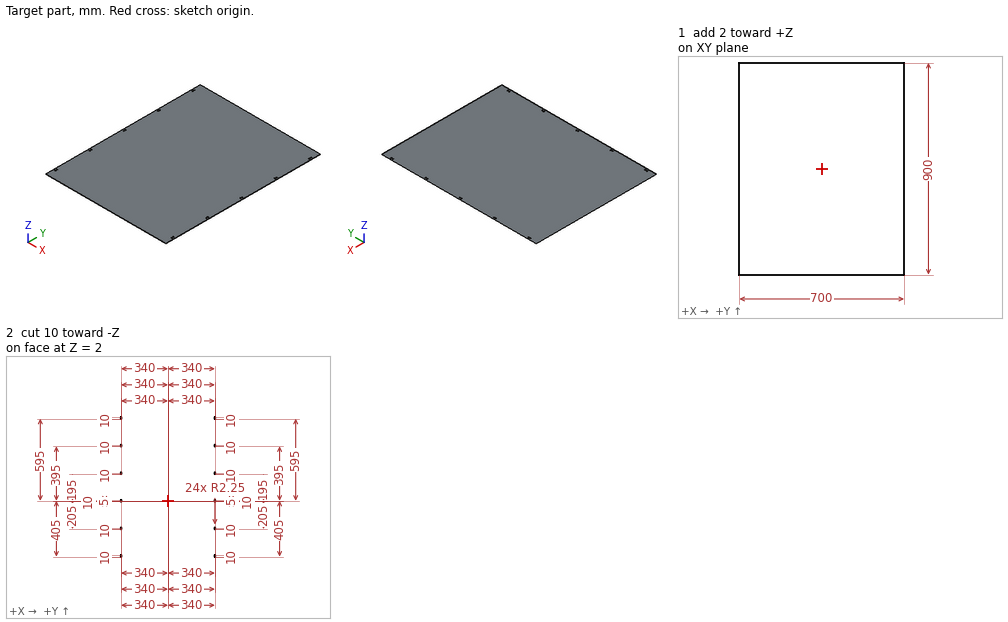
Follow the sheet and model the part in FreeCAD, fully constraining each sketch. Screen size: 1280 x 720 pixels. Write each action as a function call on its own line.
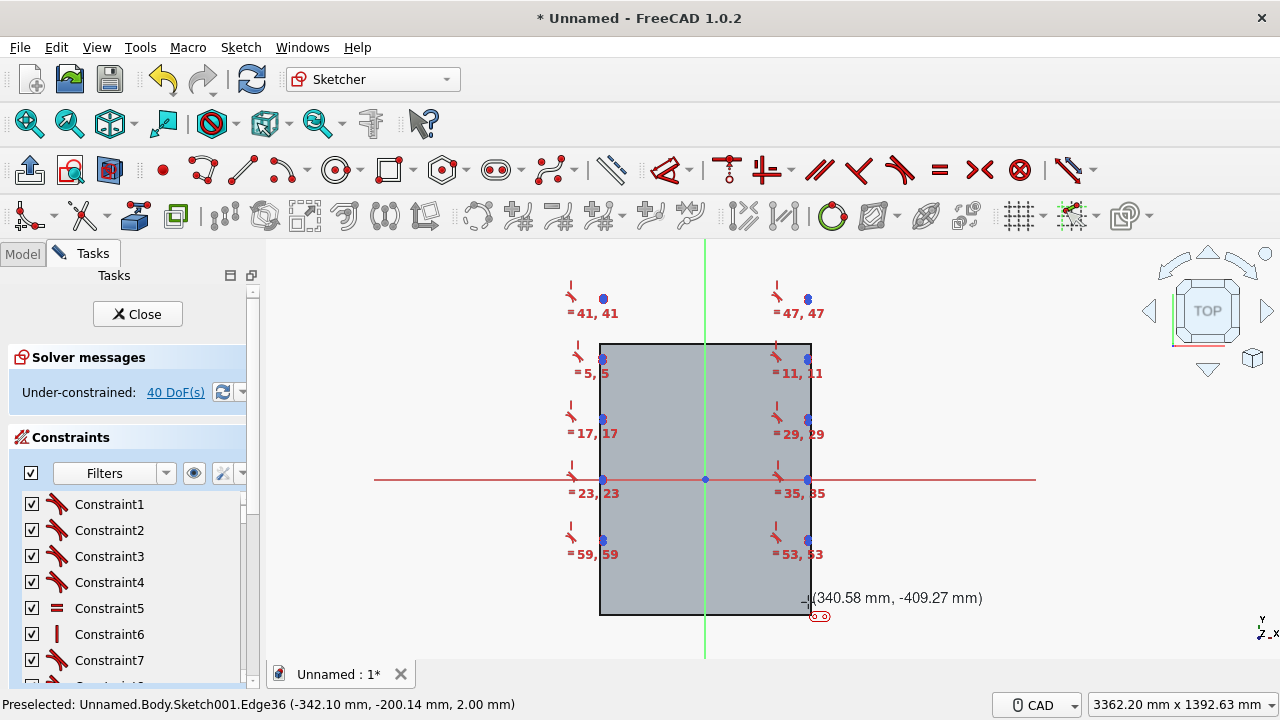
click(808, 602)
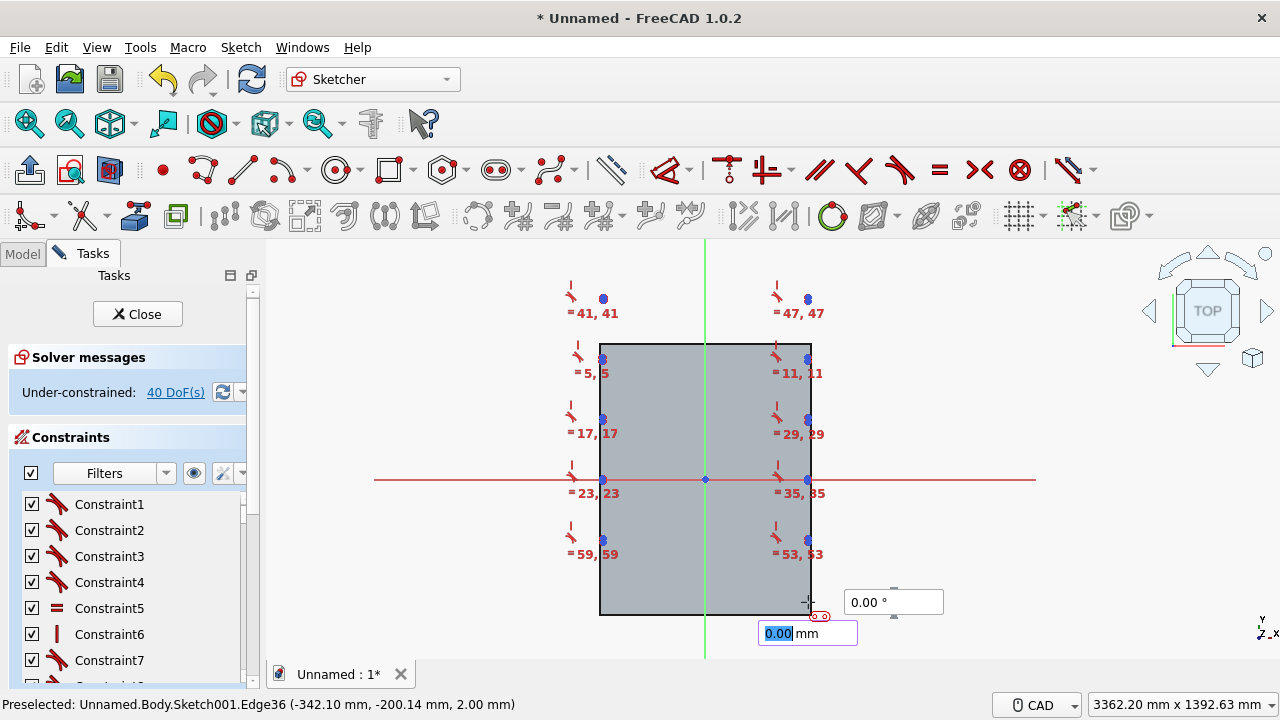
scroll(808, 599, up, 9)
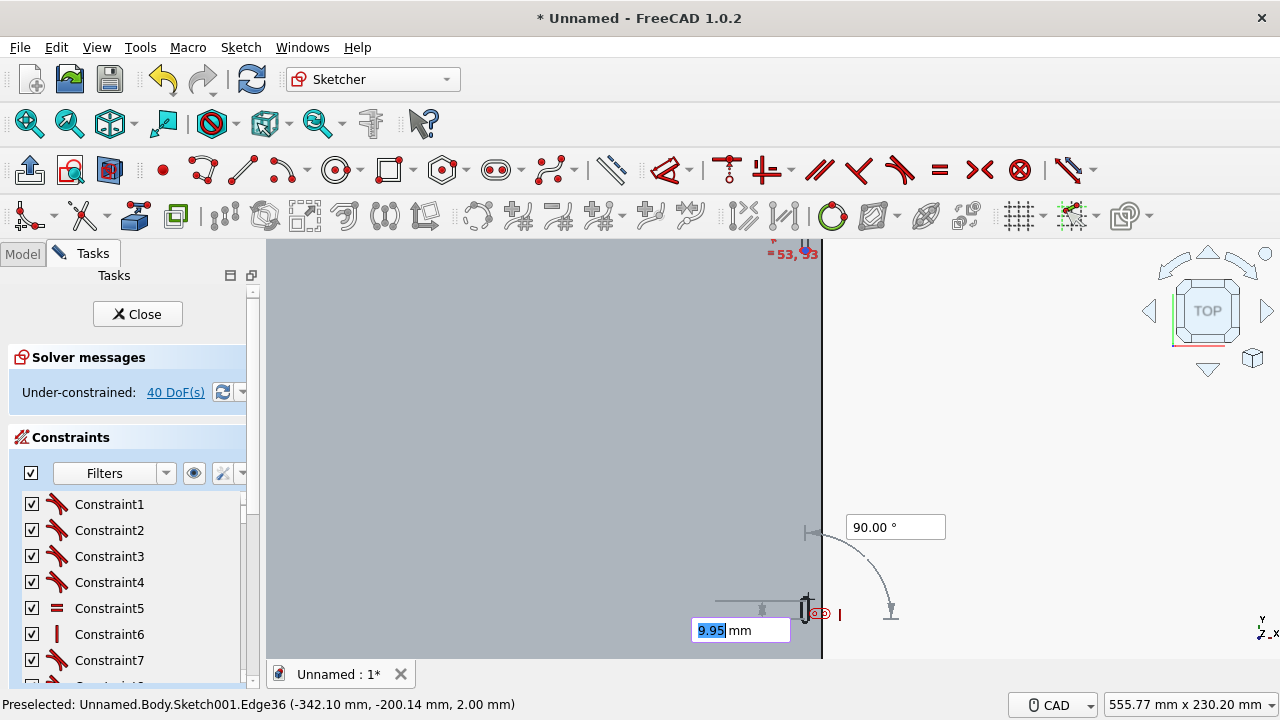
click(805, 593)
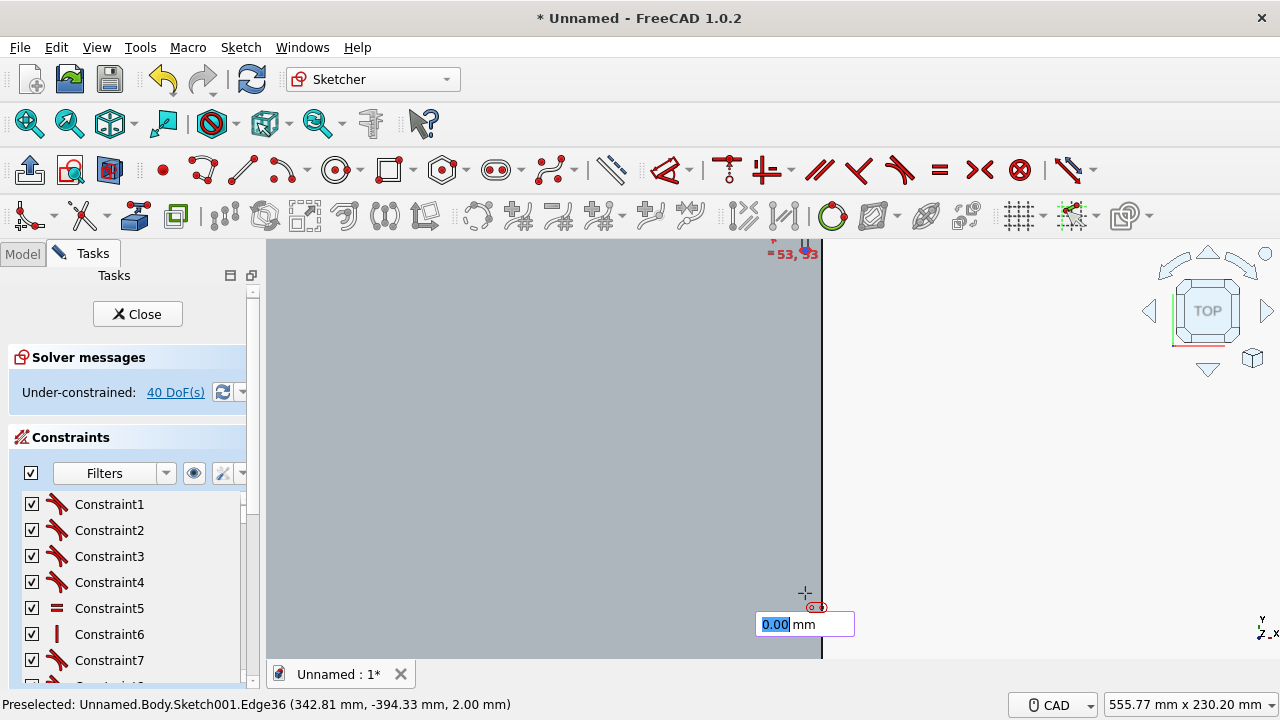
scroll(800, 602, up, 7)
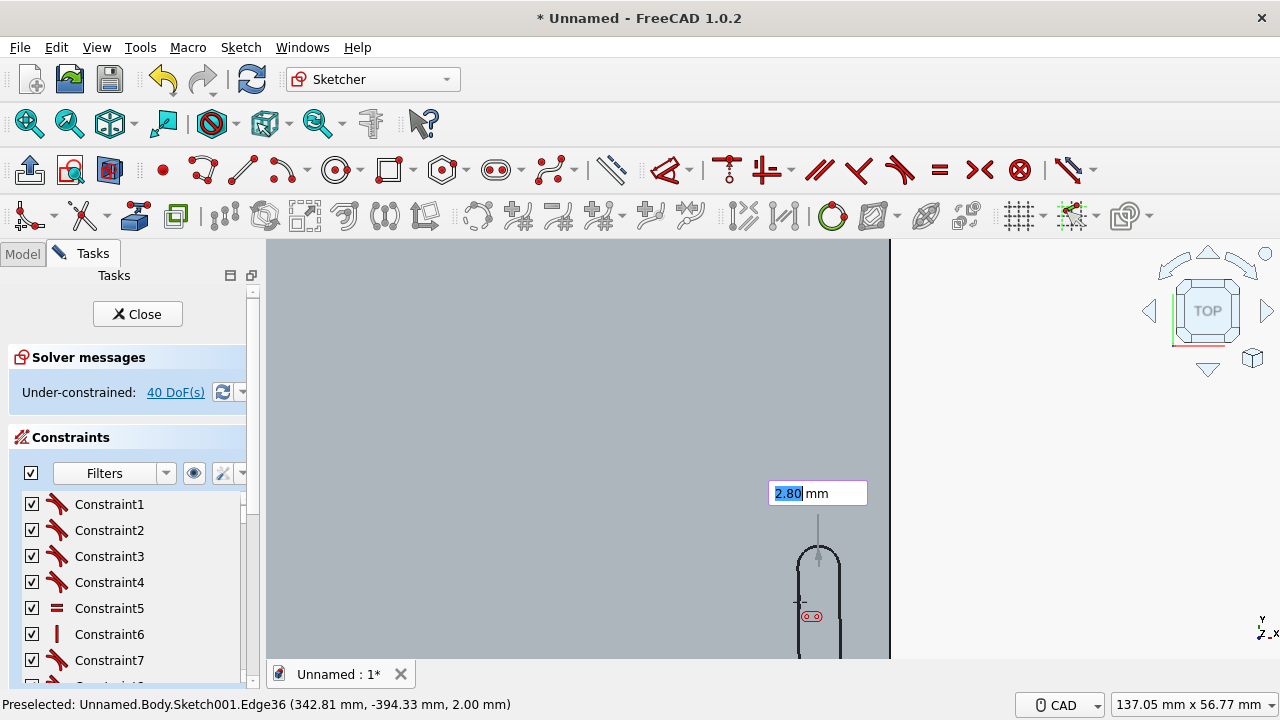
click(799, 599)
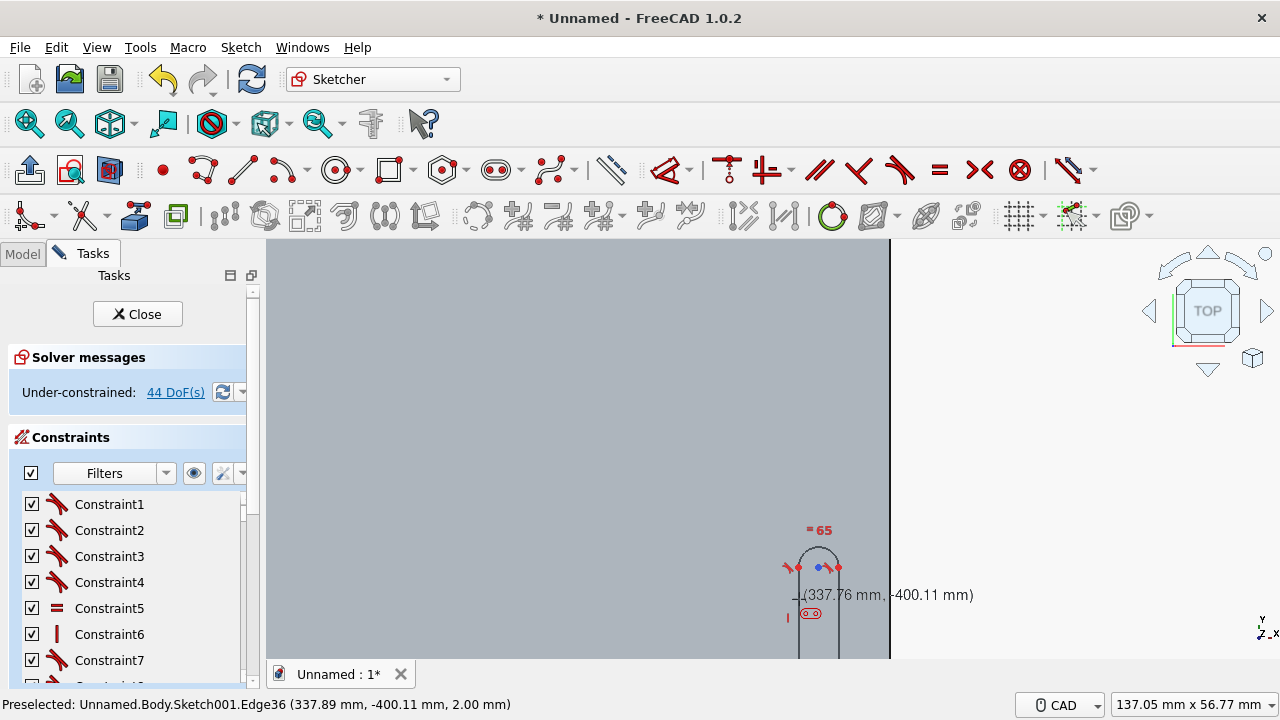
scroll(807, 600, down, 16)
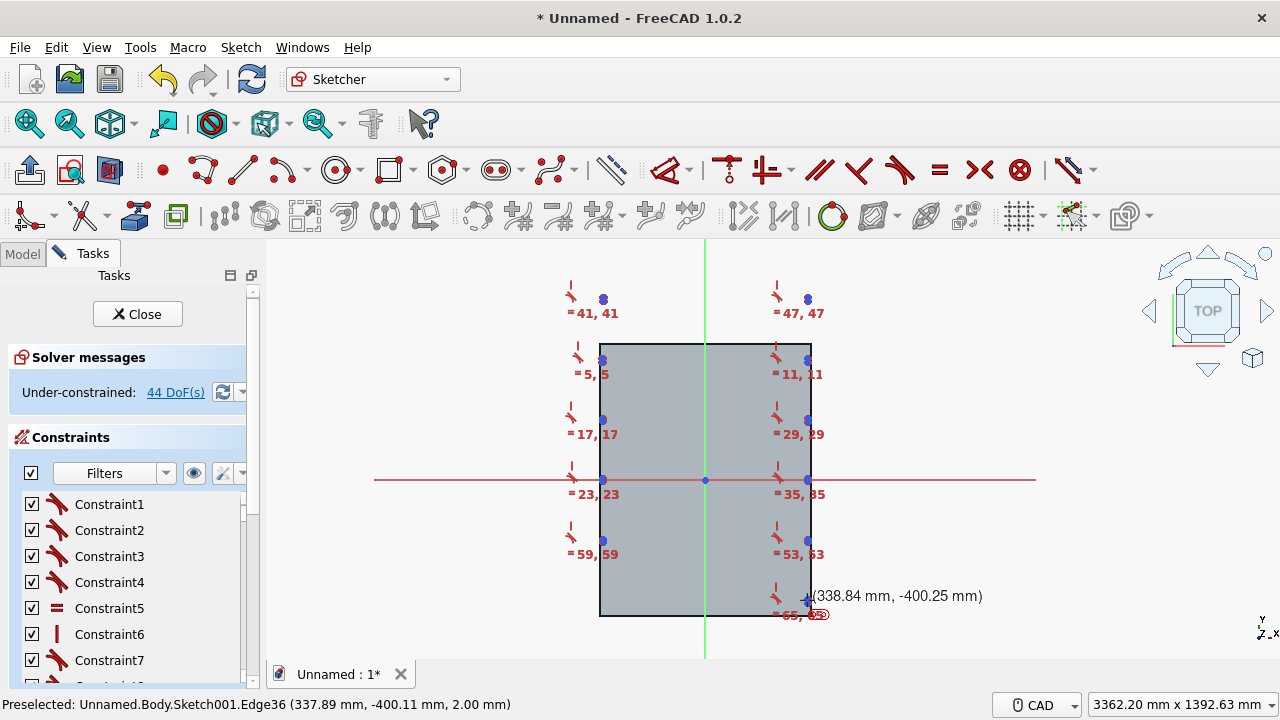
scroll(603, 602, up, 18)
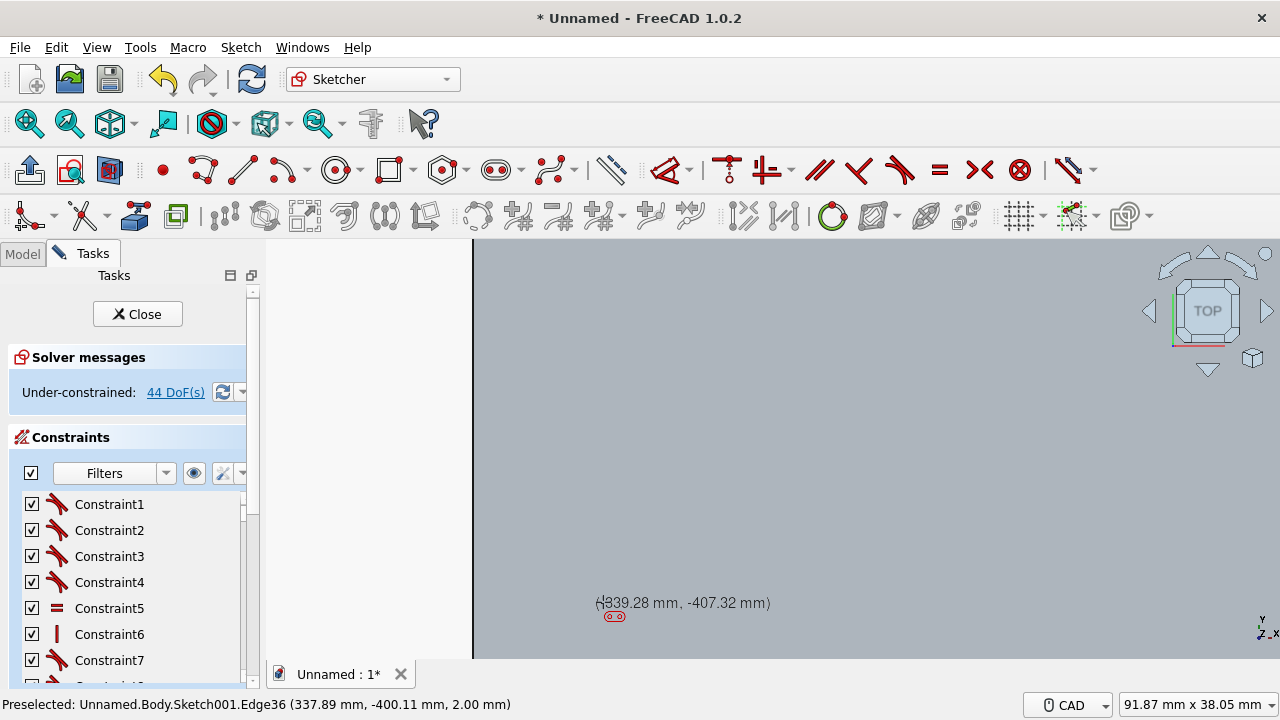
scroll(602, 602, down, 18)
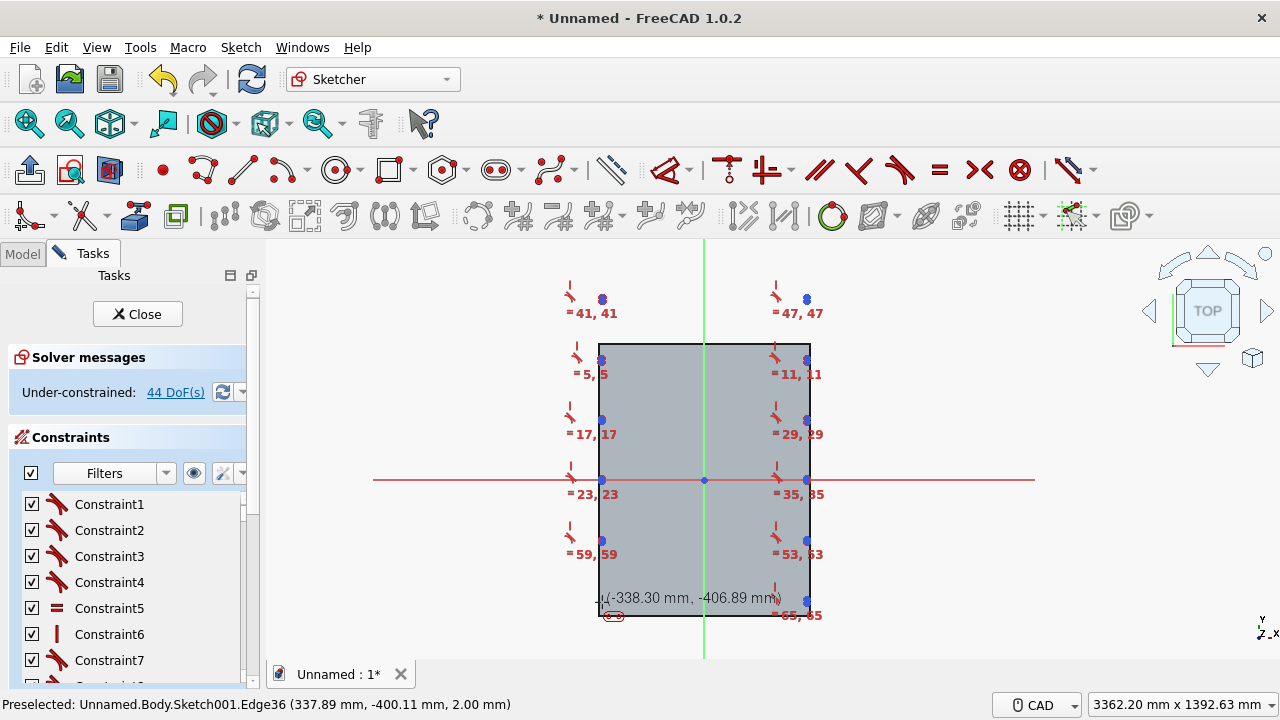
click(602, 602)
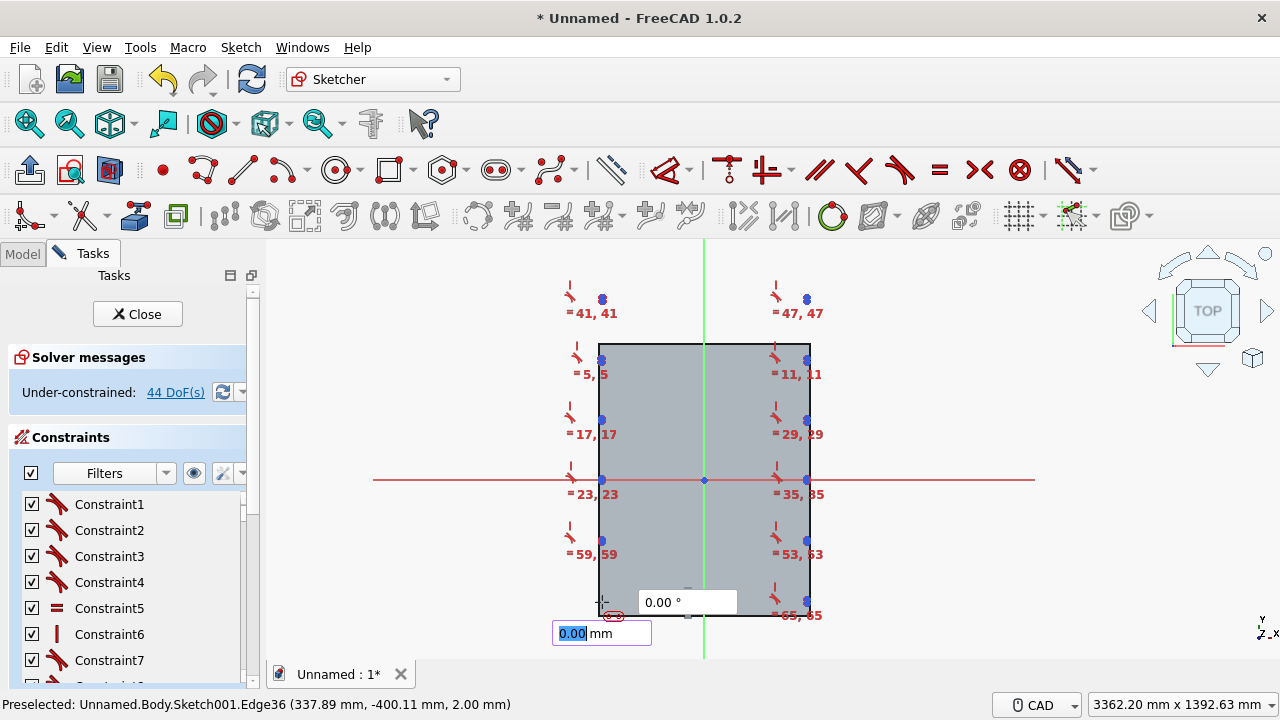
scroll(602, 599, up, 9)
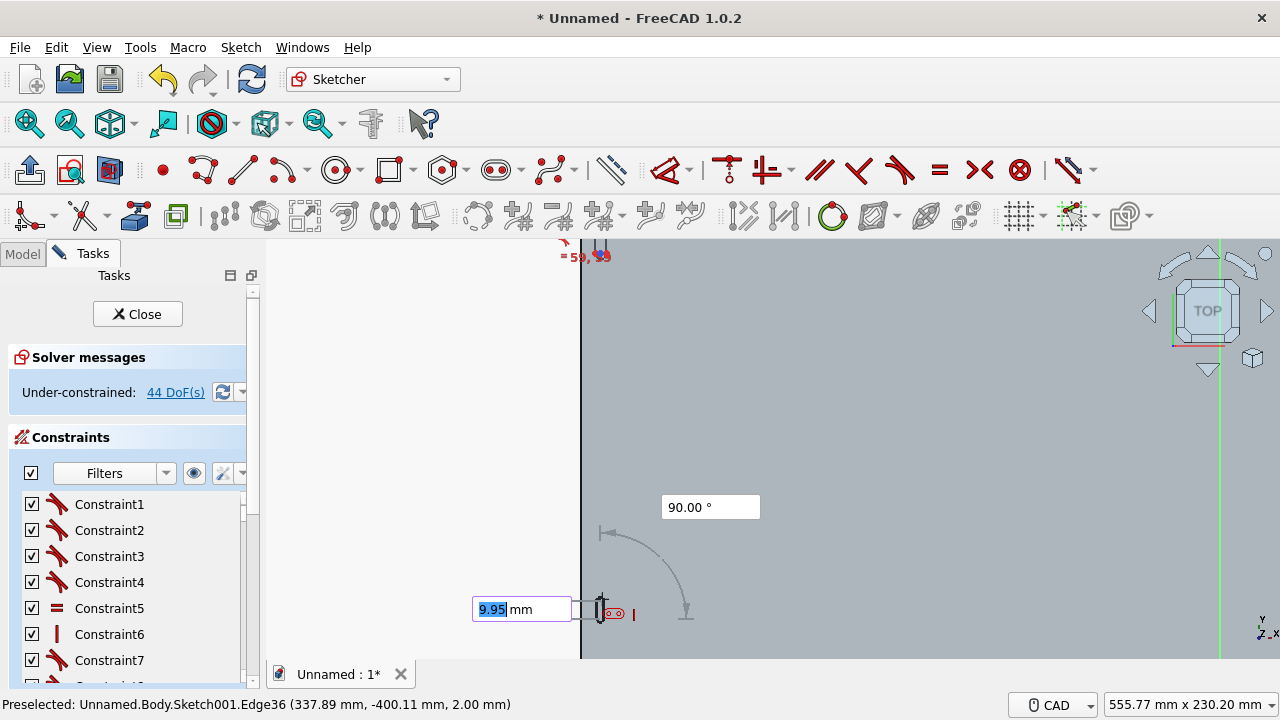
click(600, 596)